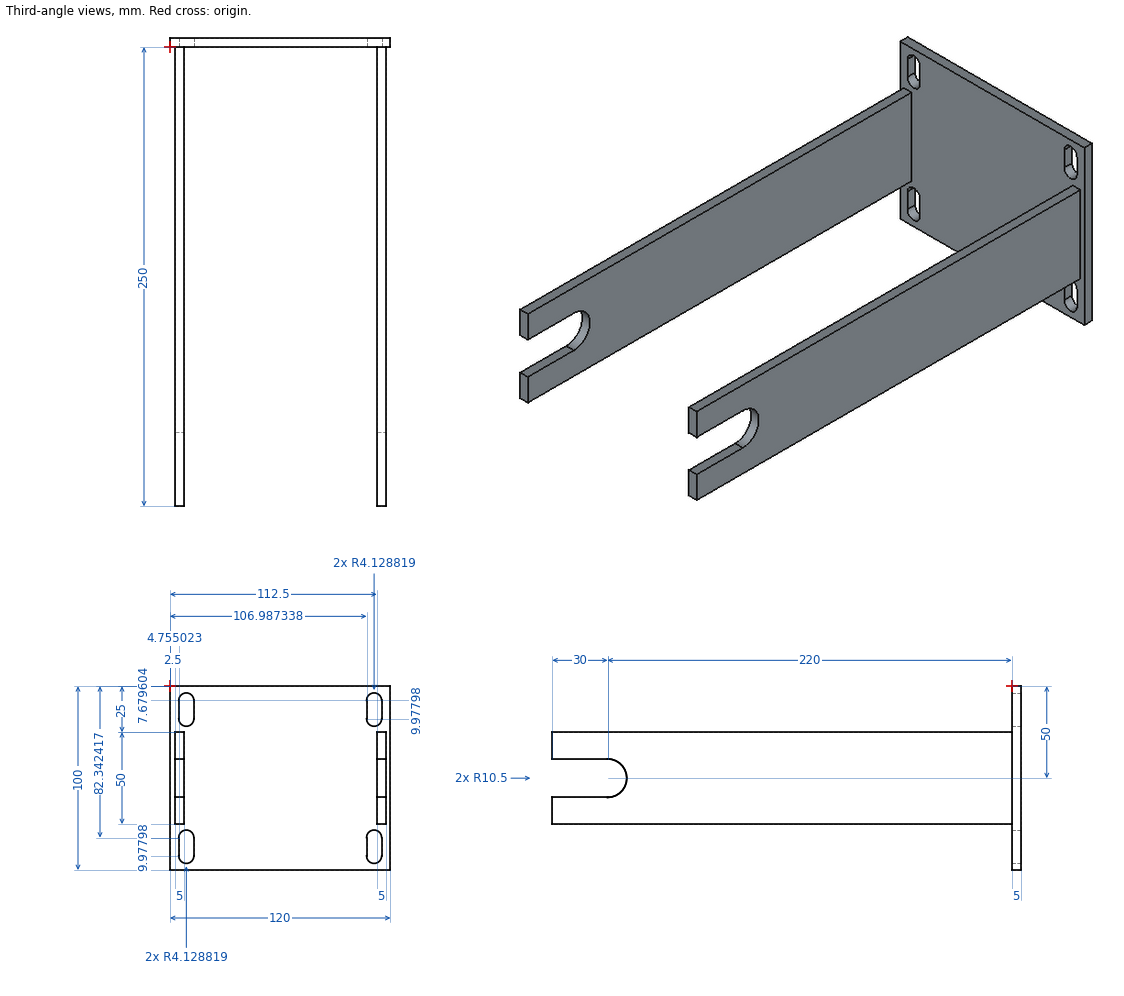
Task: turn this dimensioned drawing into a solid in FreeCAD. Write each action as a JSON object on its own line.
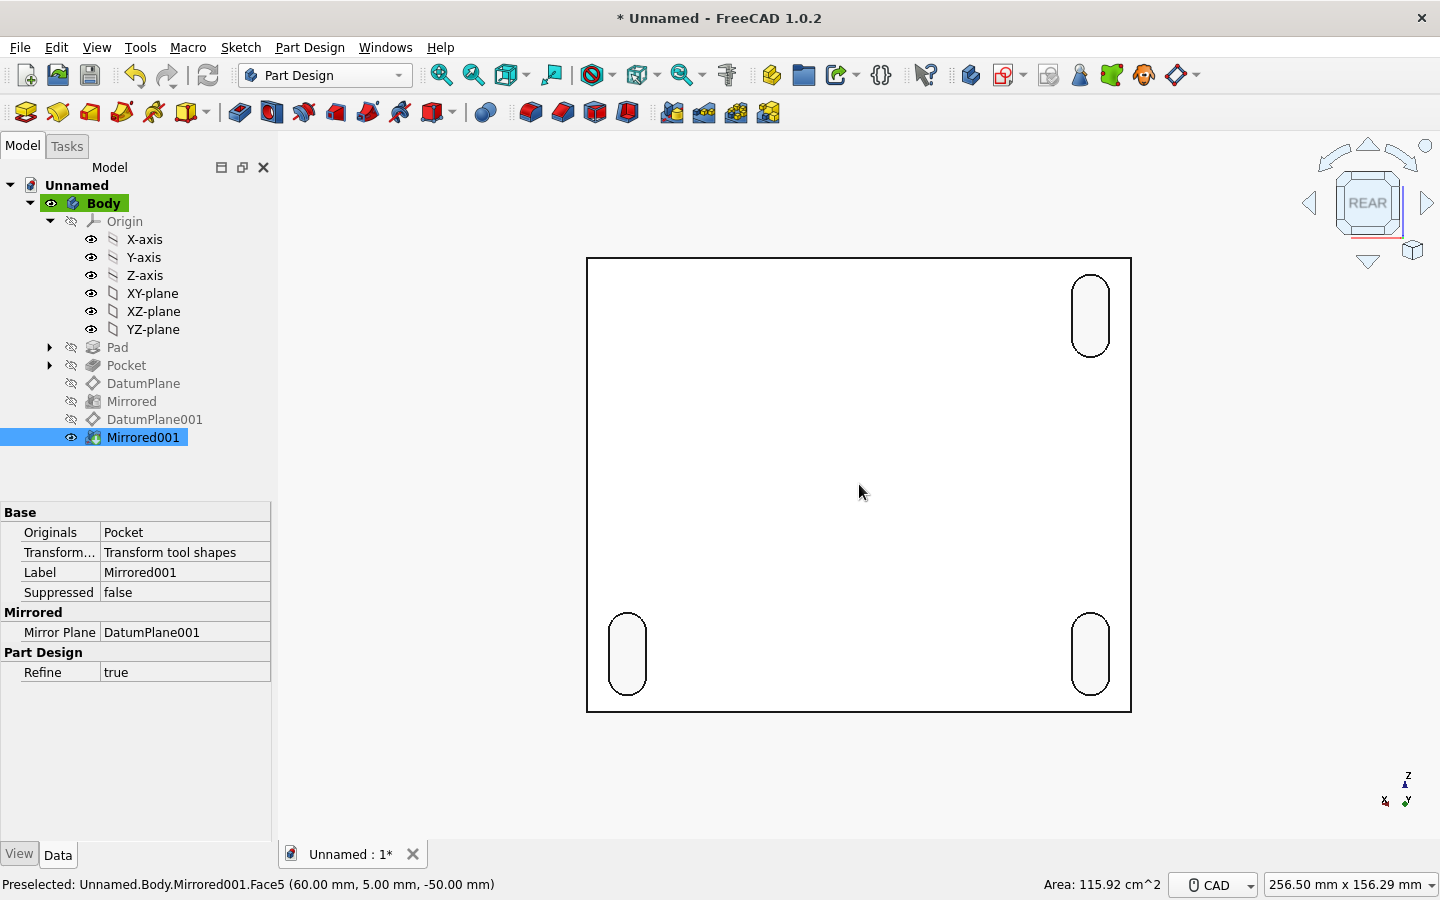
{"action": "left_click", "coordinate": [1004, 76]}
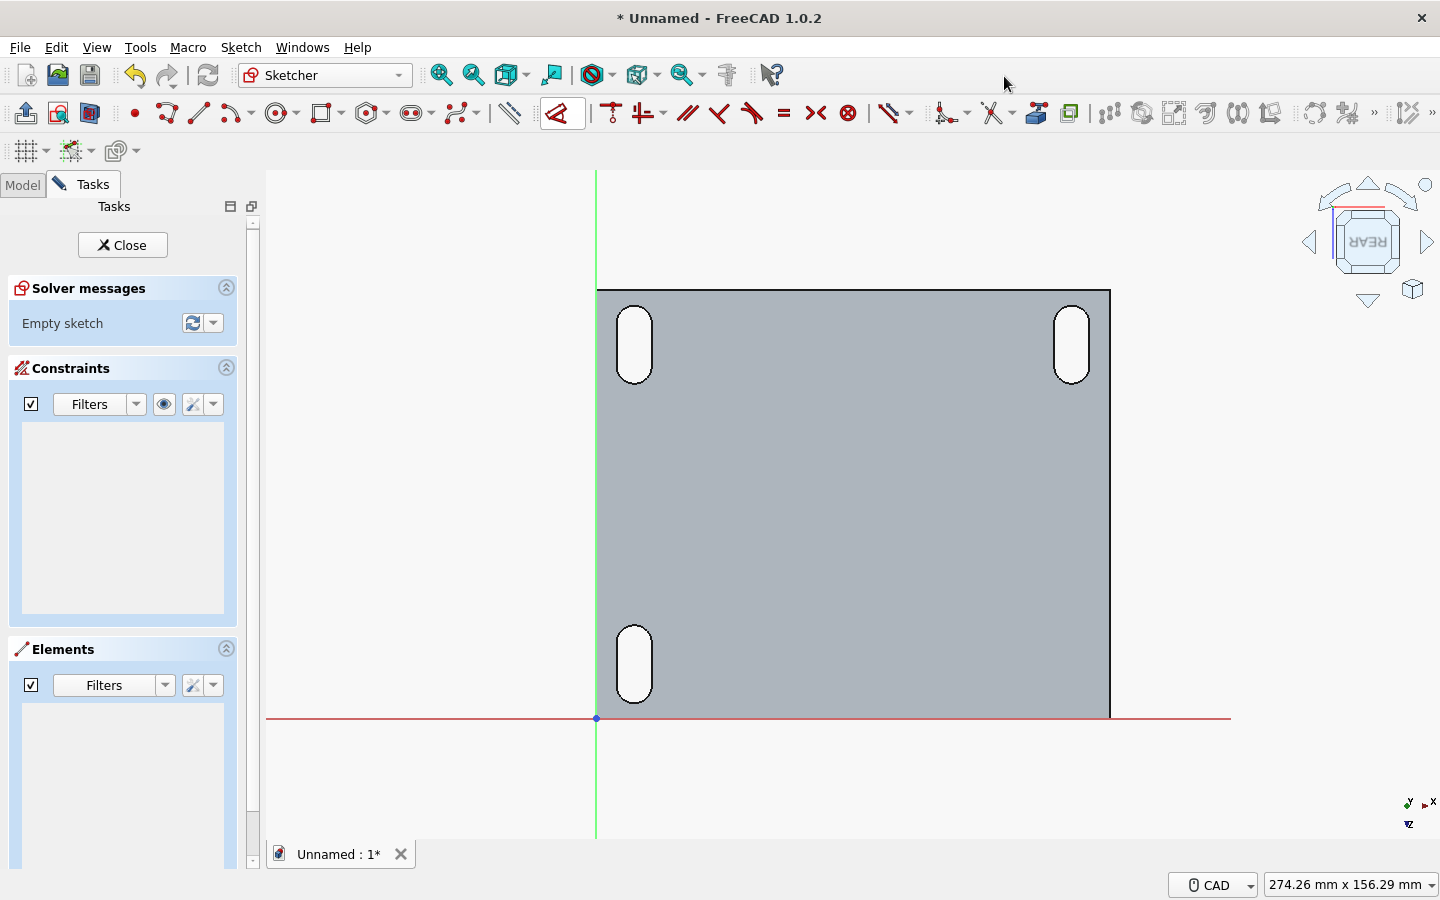
{"action": "scroll", "coordinate": [1129, 696], "scroll_direction": "up", "scroll_amount": 9}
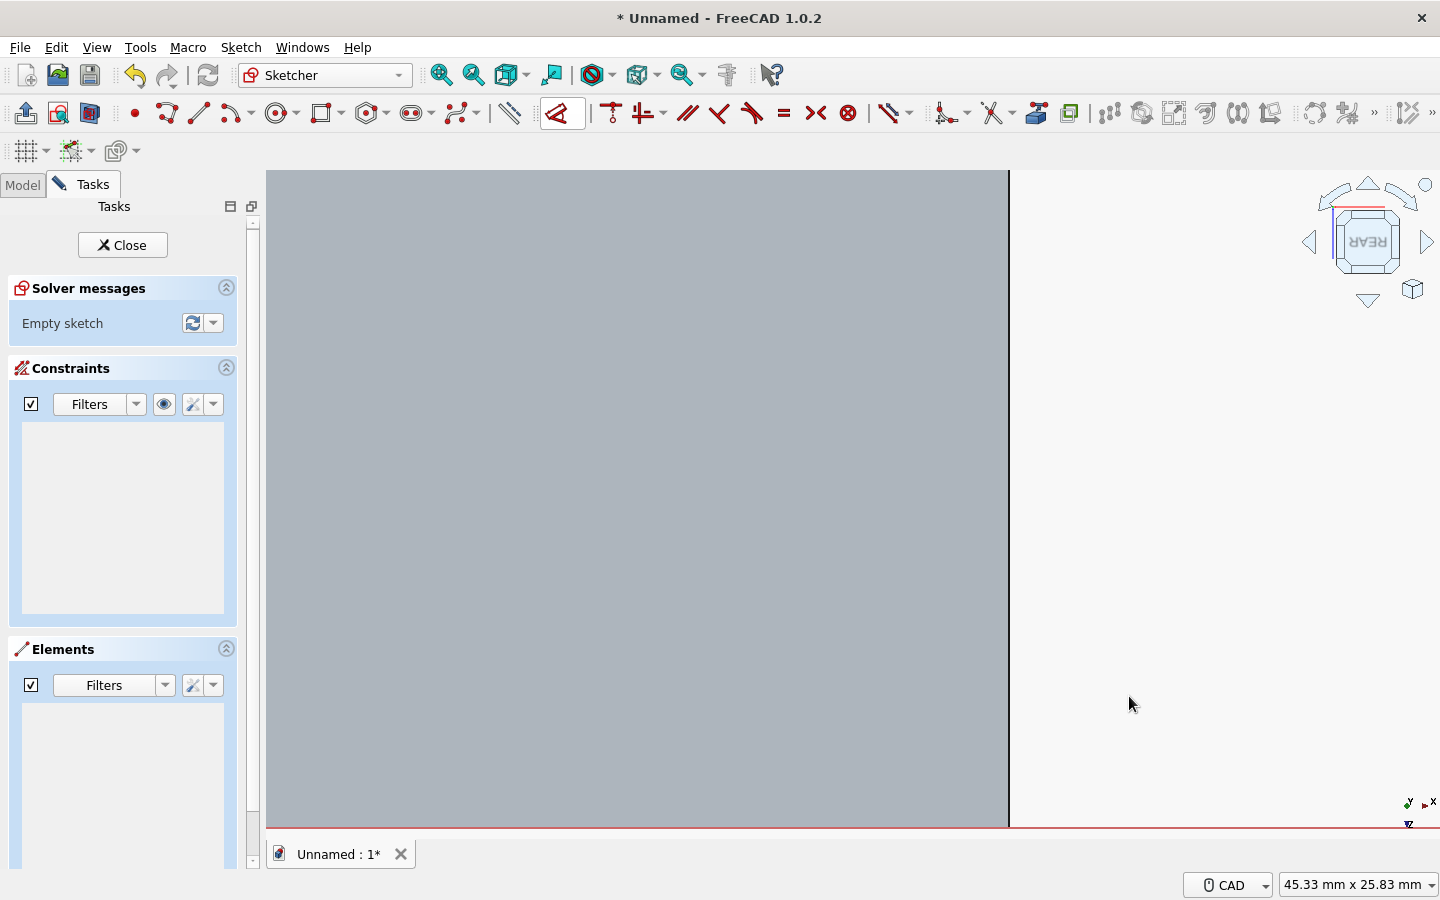
{"action": "key", "text": "g s"}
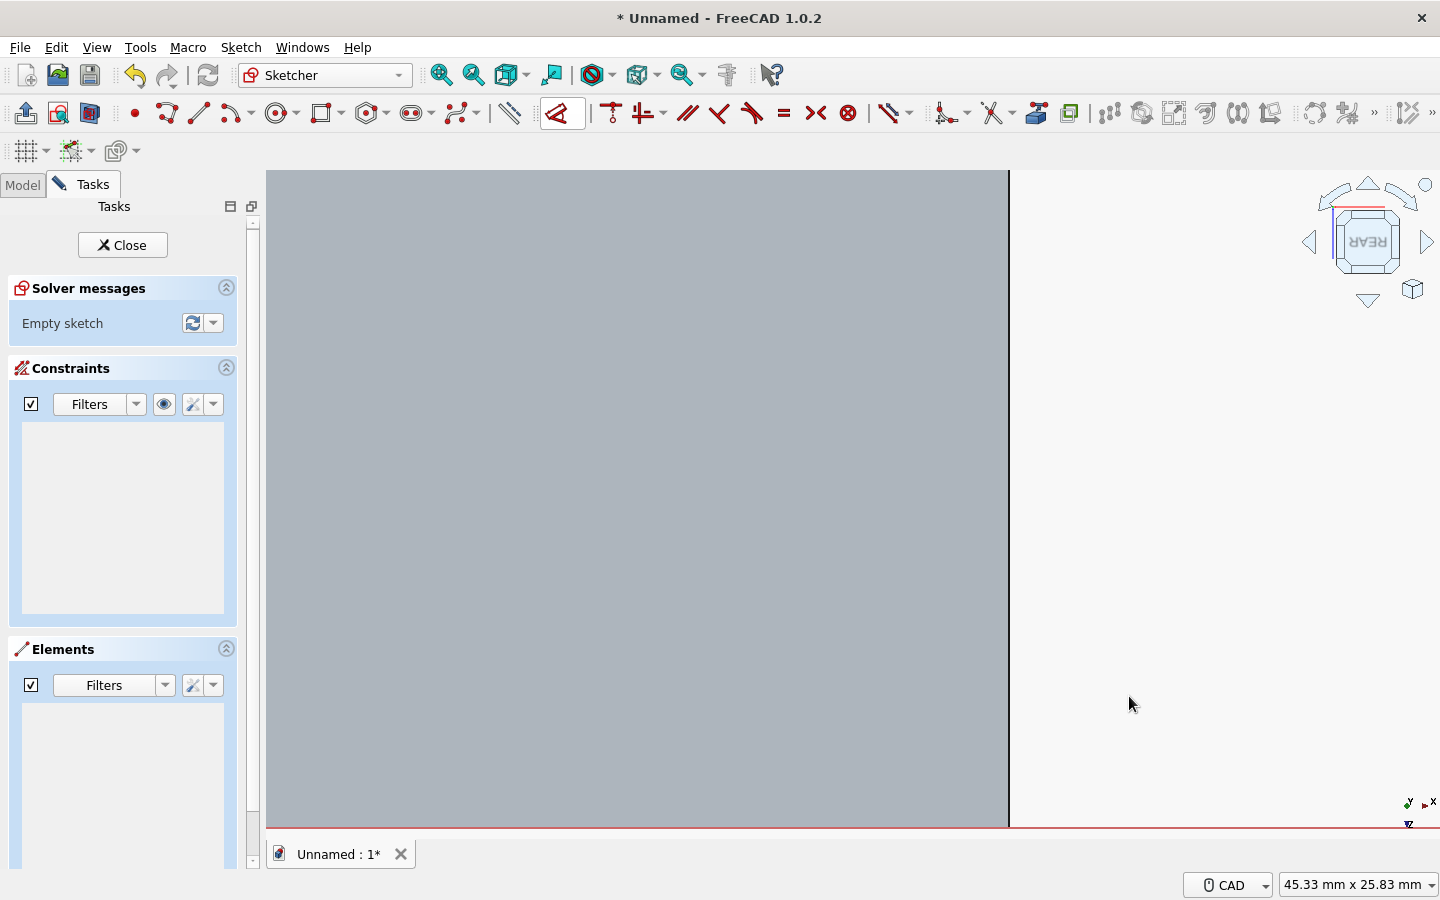
{"action": "left_click", "coordinate": [779, 629]}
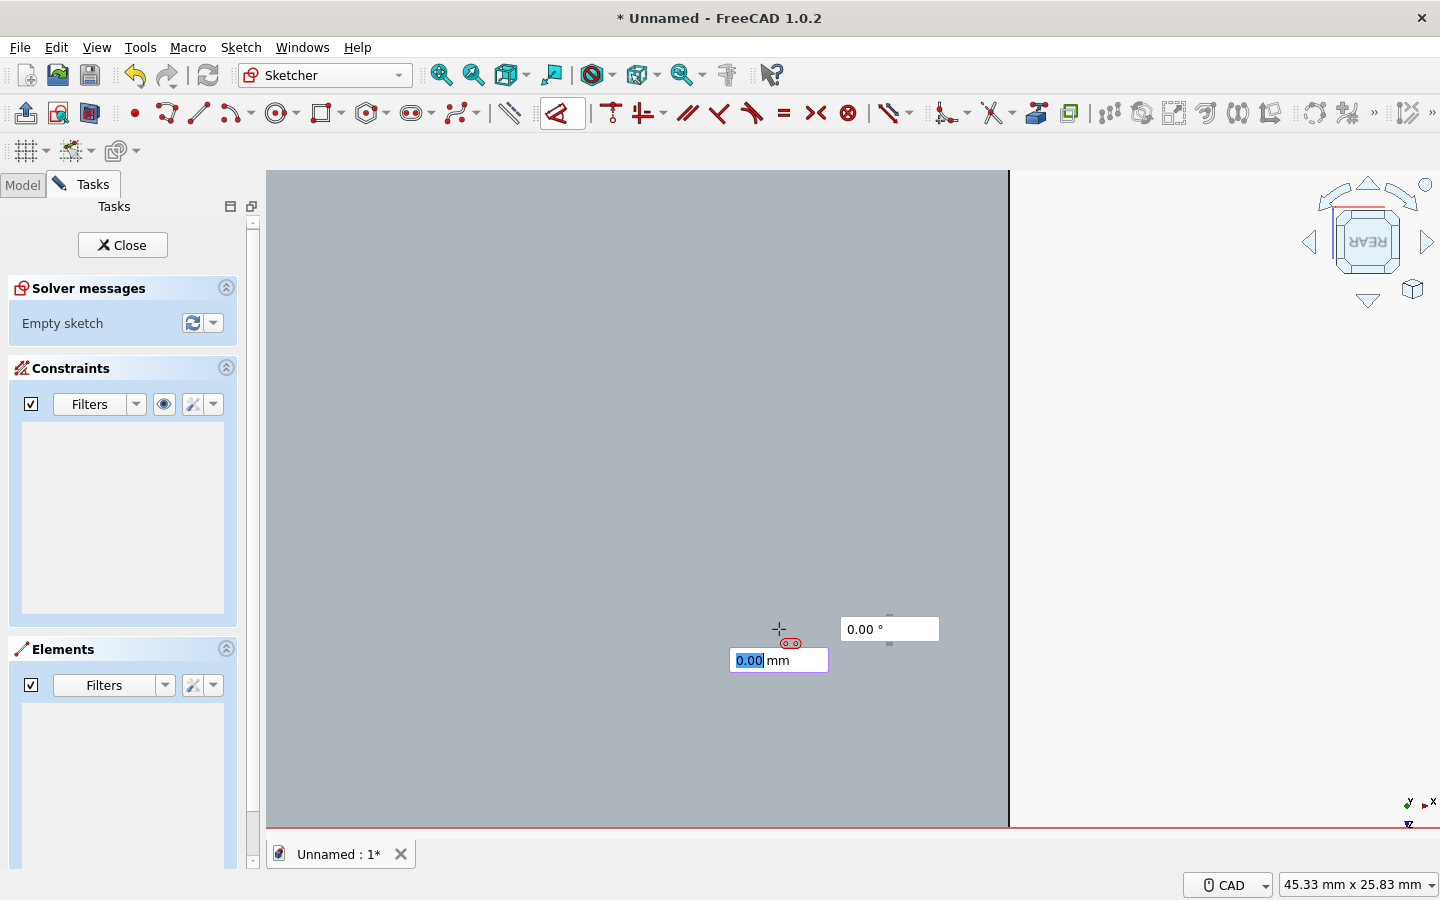
{"action": "left_click", "coordinate": [779, 371]}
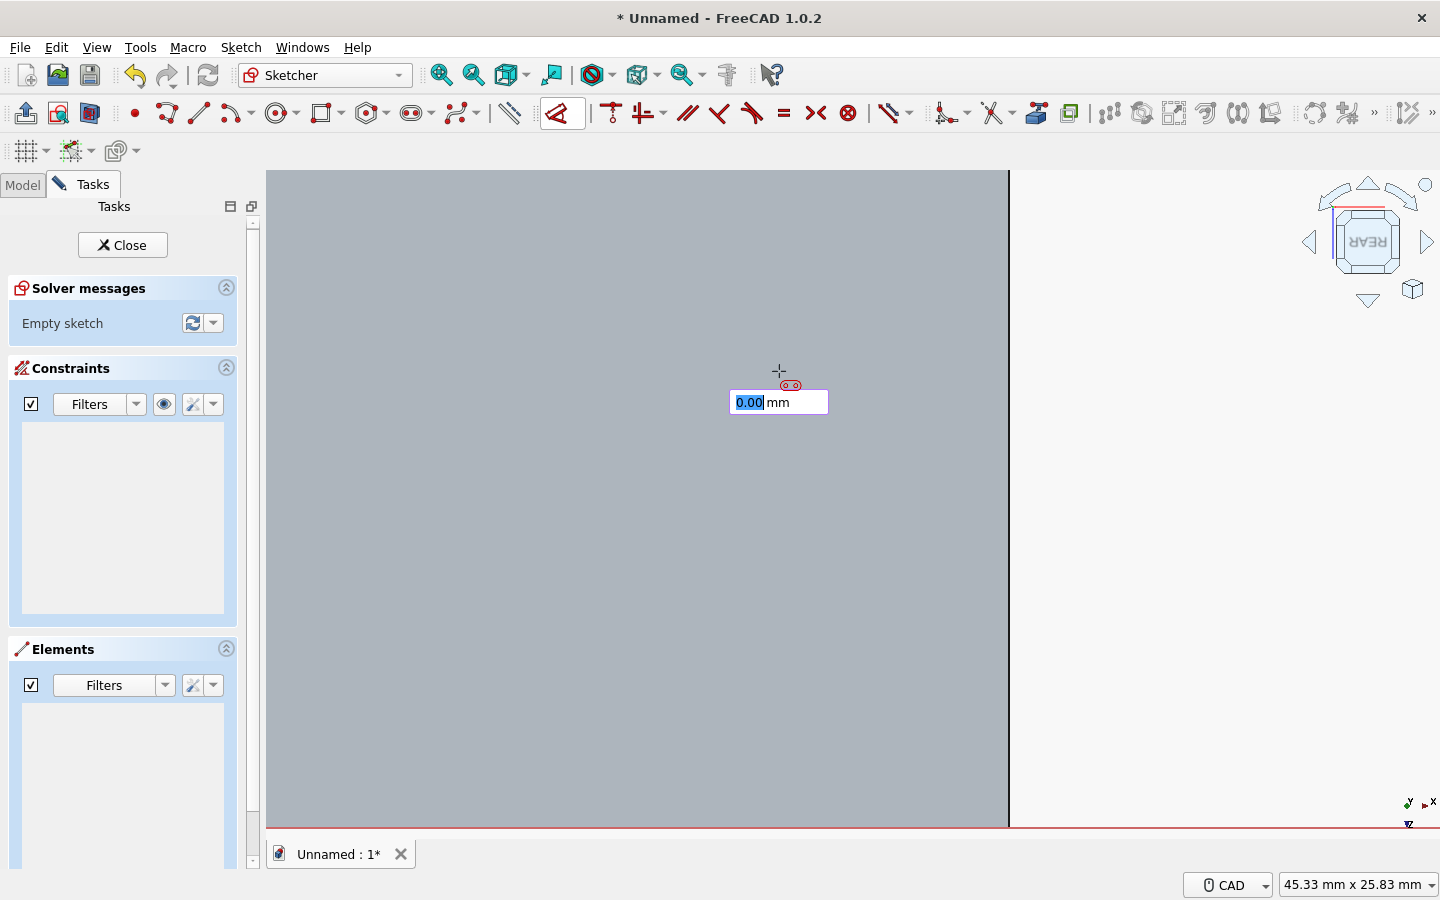
{"action": "left_click", "coordinate": [672, 500]}
{"action": "key", "text": "Escape"}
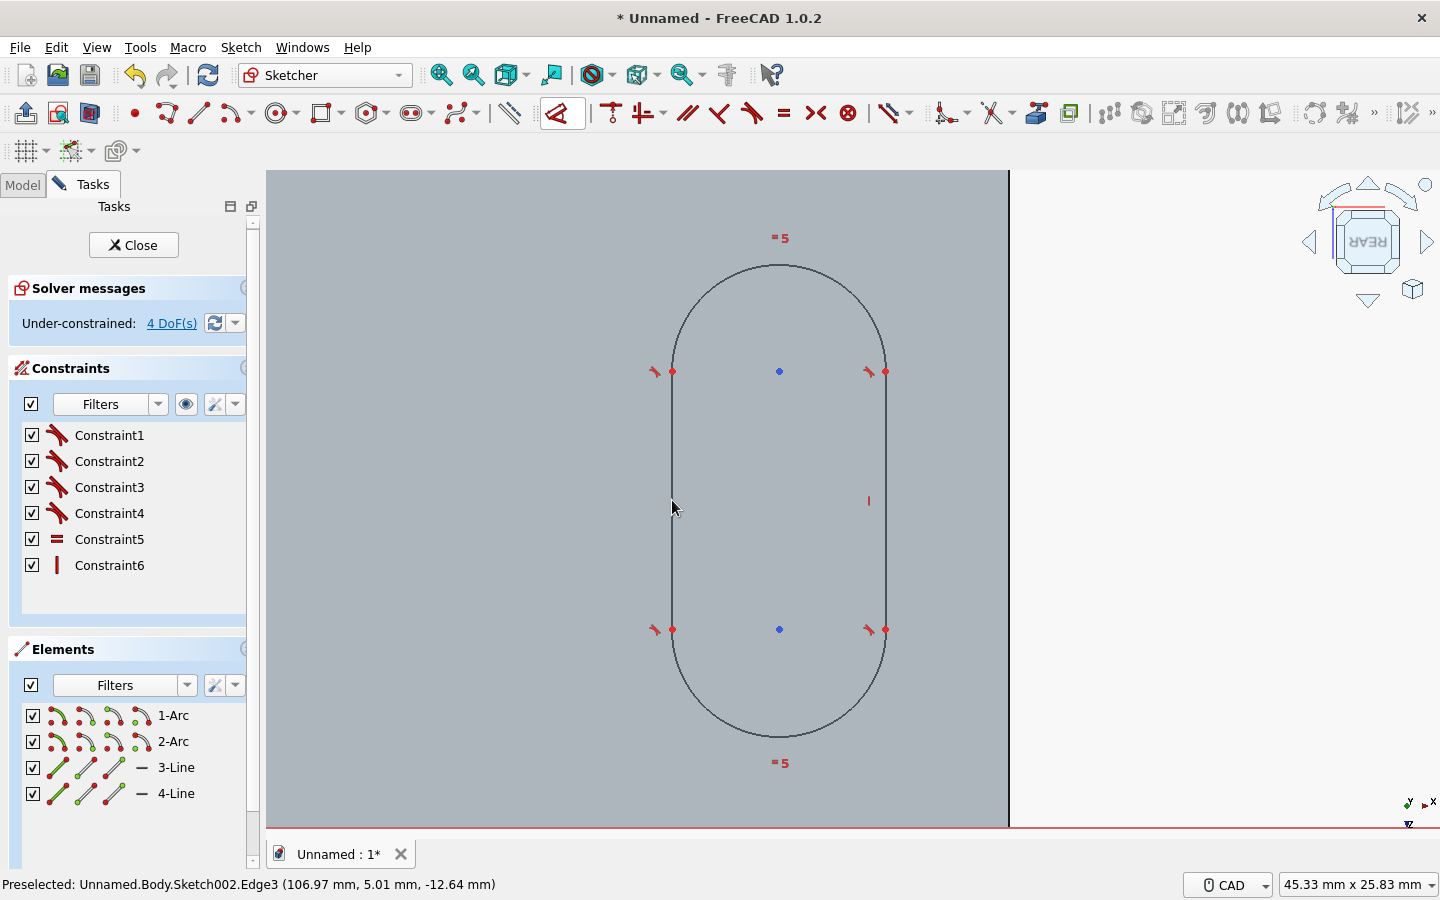
{"action": "left_click", "coordinate": [716, 717]}